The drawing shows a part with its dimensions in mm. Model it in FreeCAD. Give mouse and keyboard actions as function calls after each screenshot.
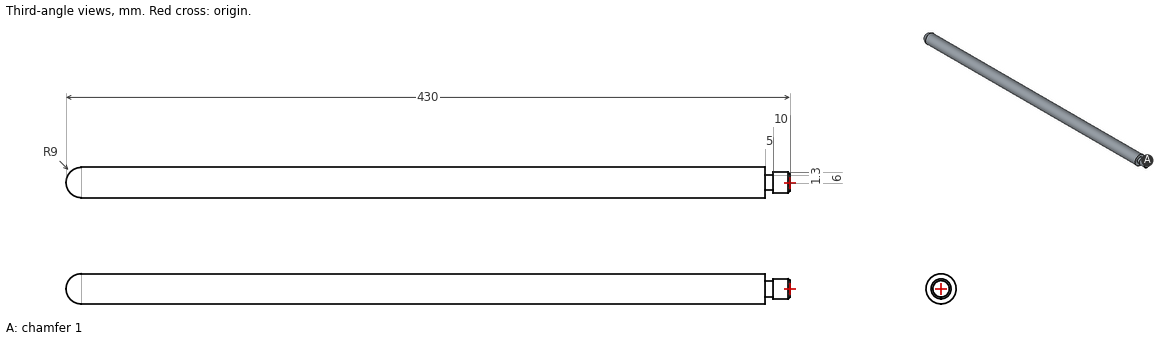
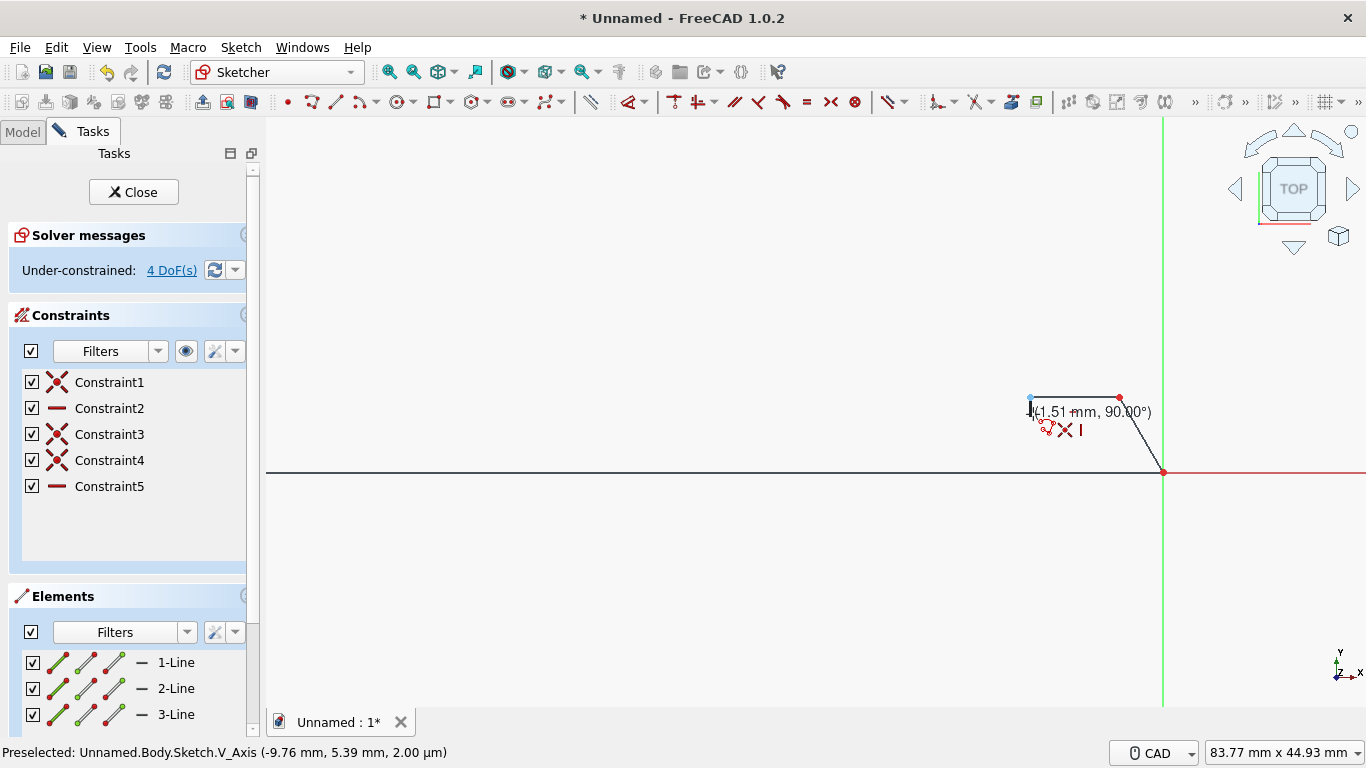
click(1030, 411)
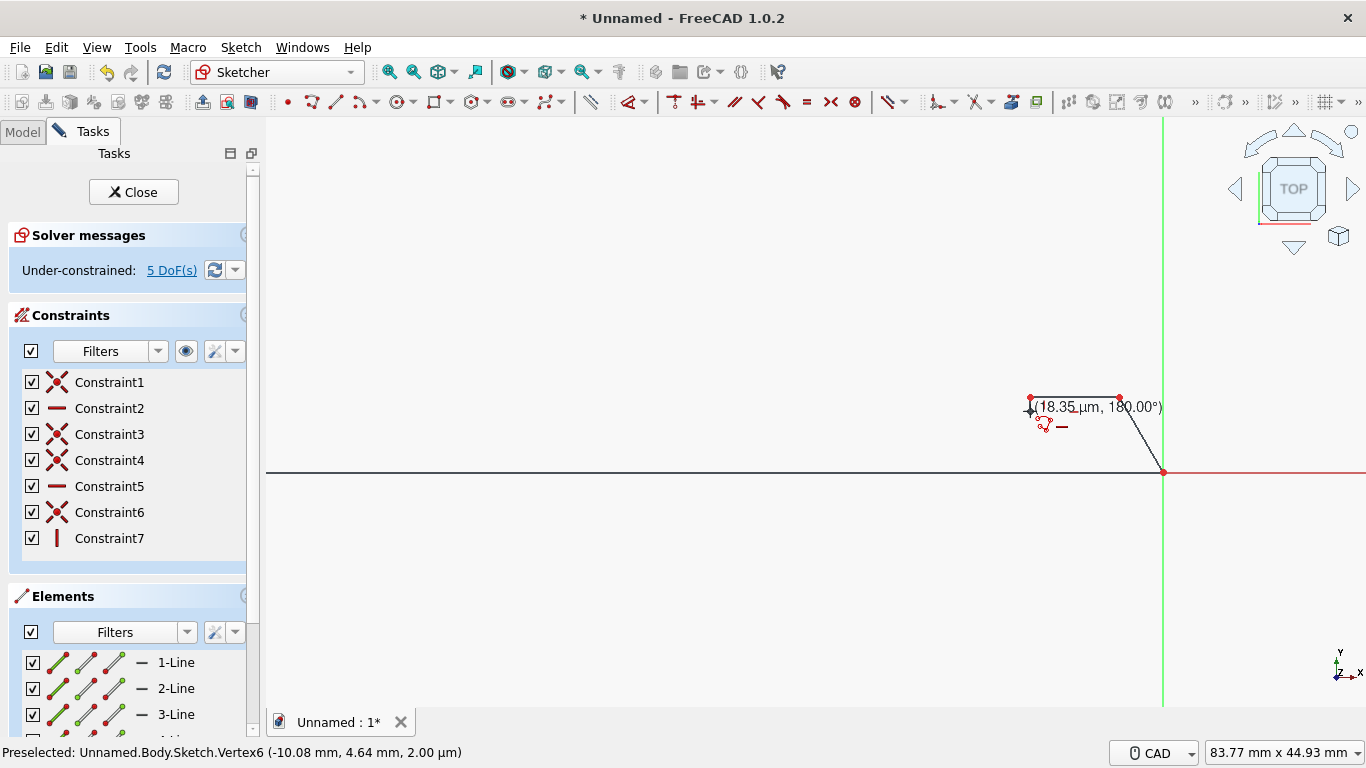
scroll(1047, 412, down, 11)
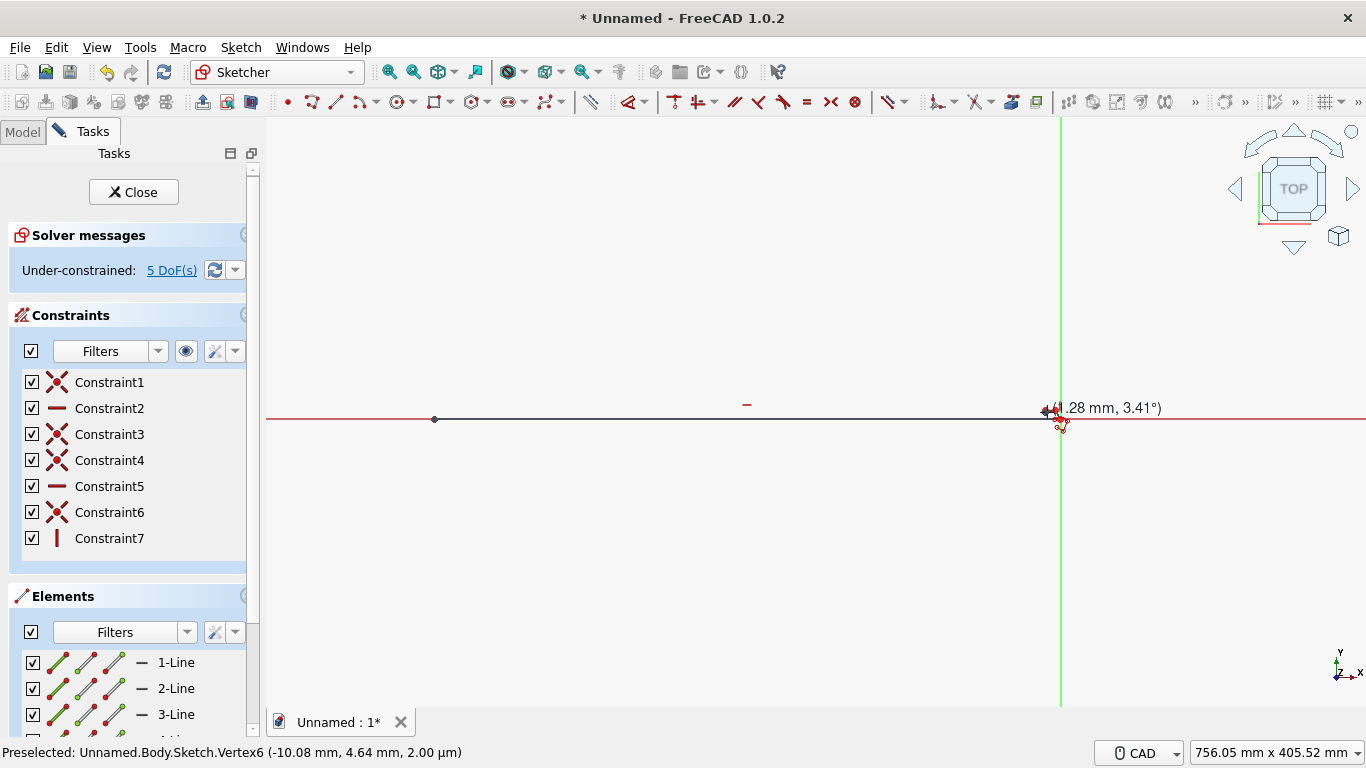
scroll(1039, 412, up, 5)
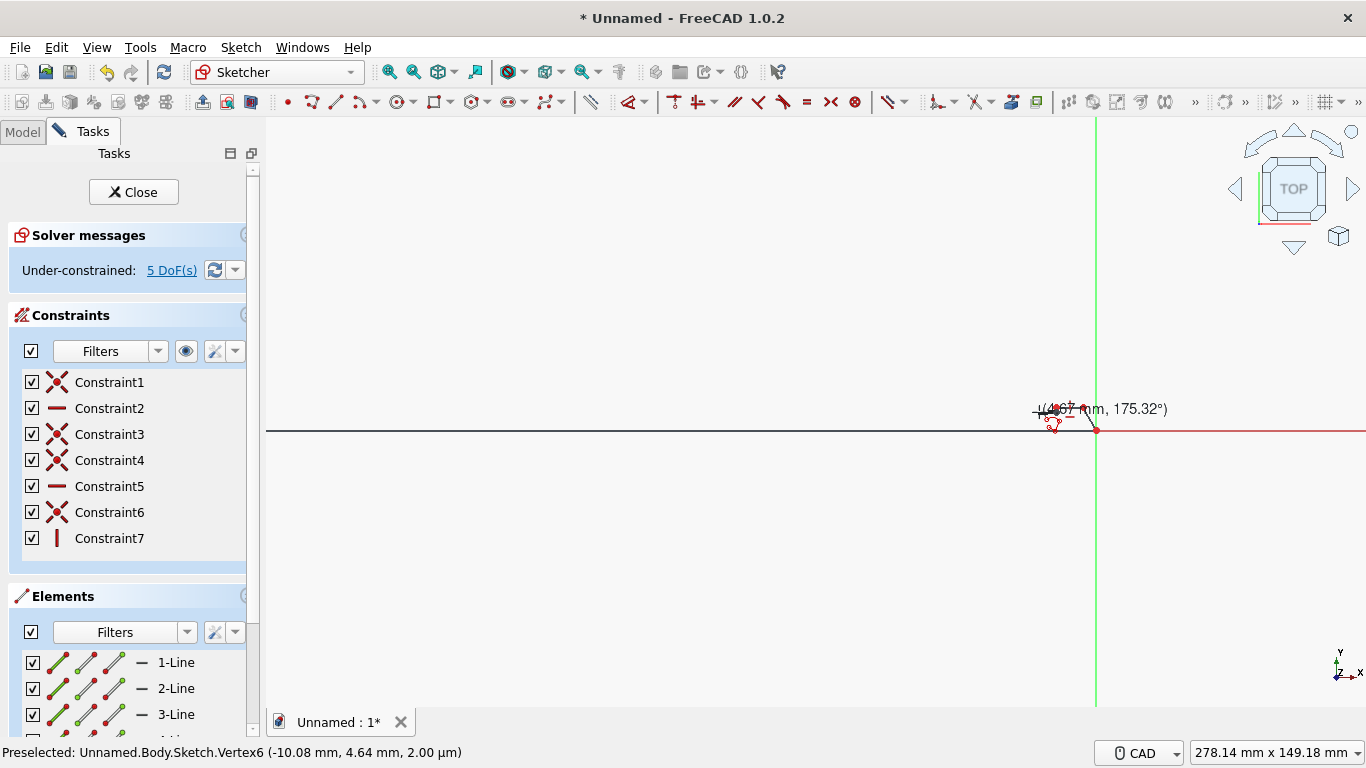
click(1037, 412)
click(1037, 395)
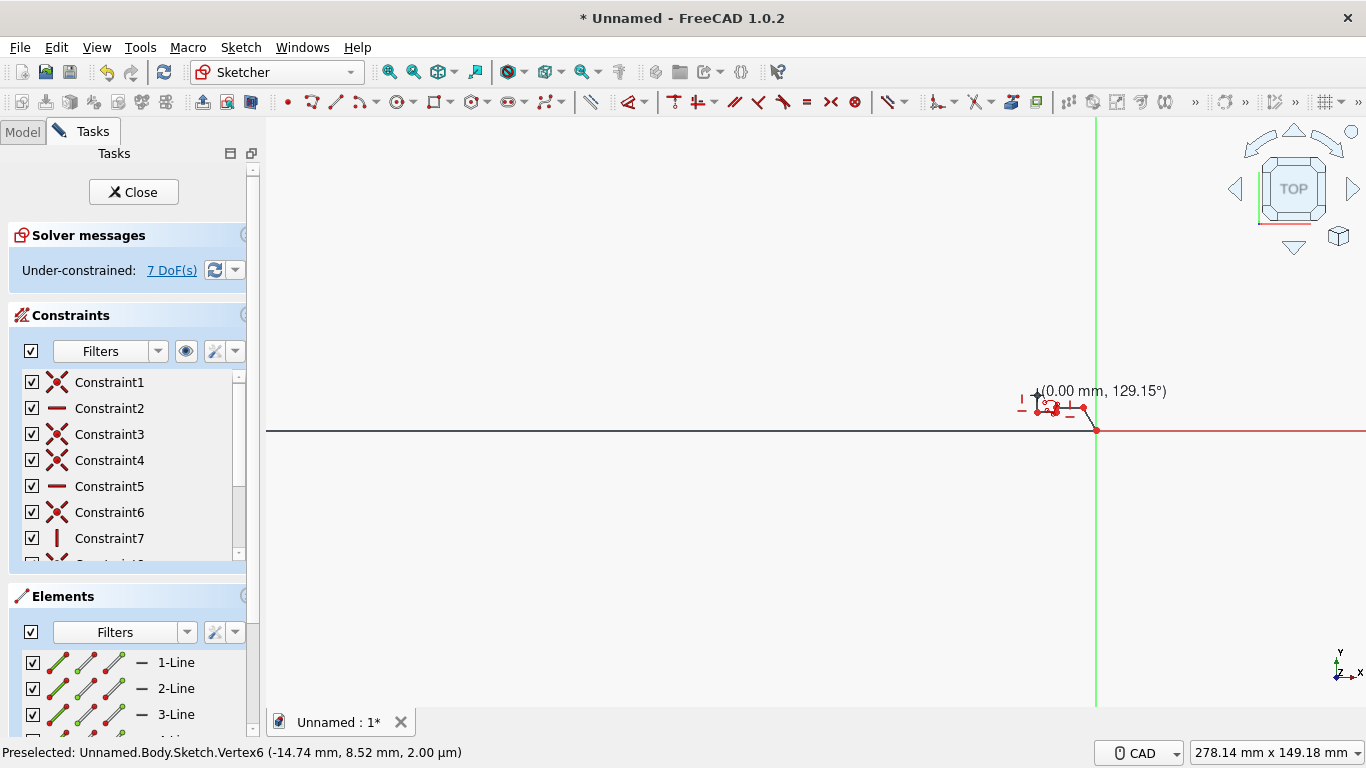
scroll(1039, 411, down, 5)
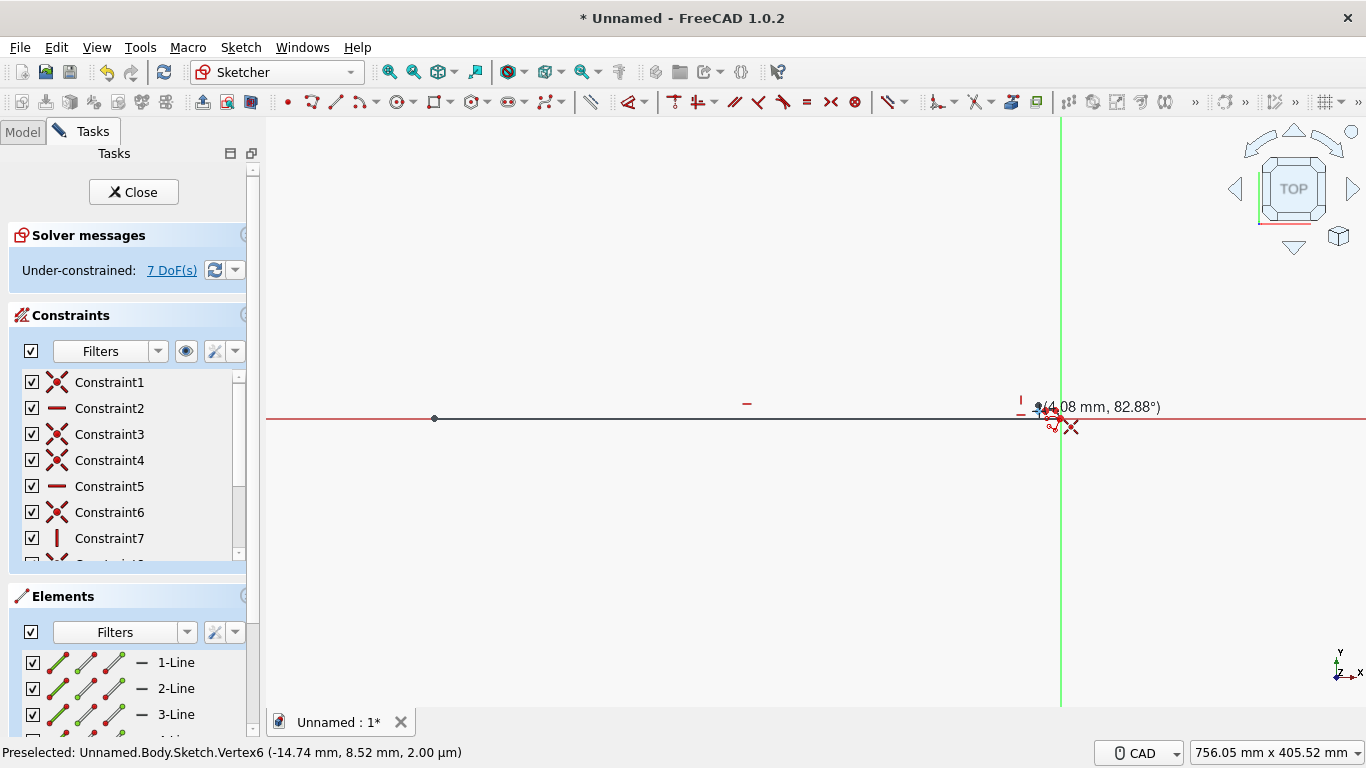
click(448, 405)
right_click(448, 405)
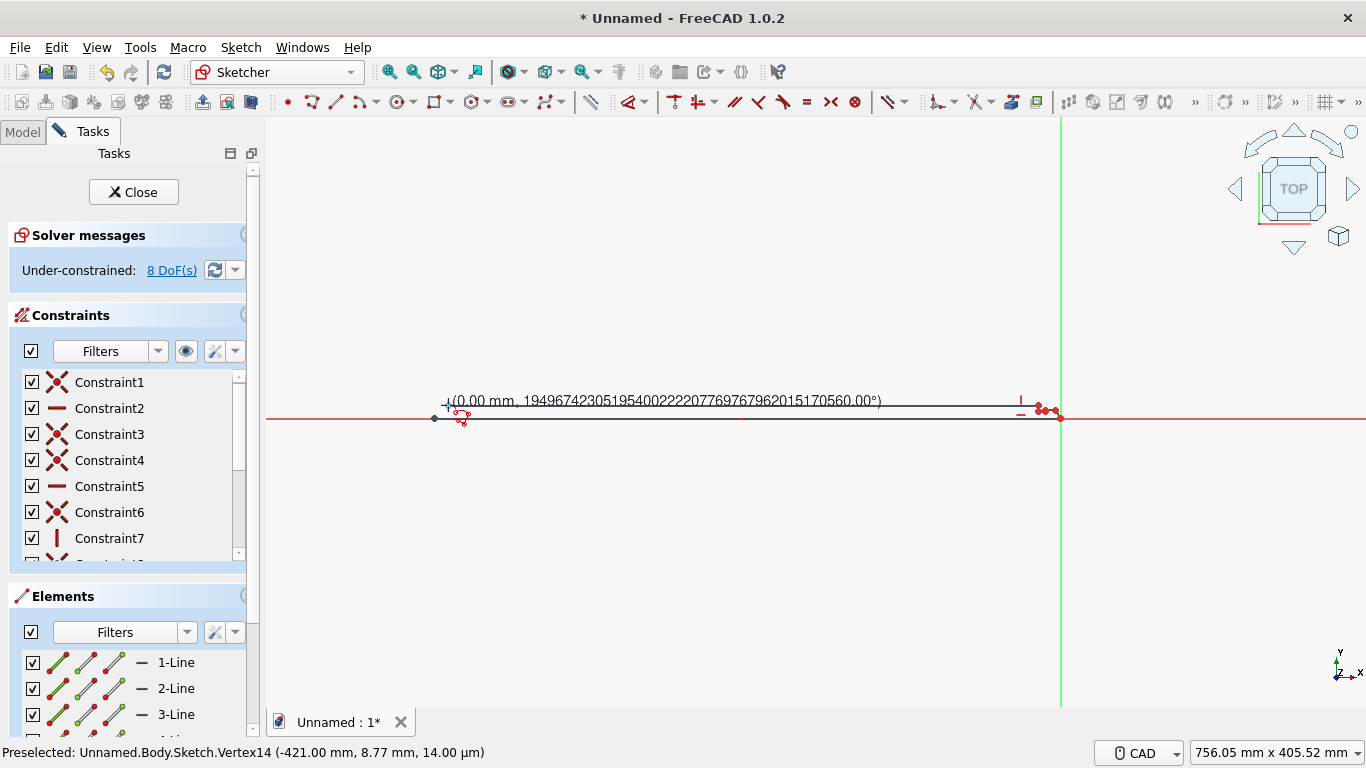
key(g)
key(3)
key(a)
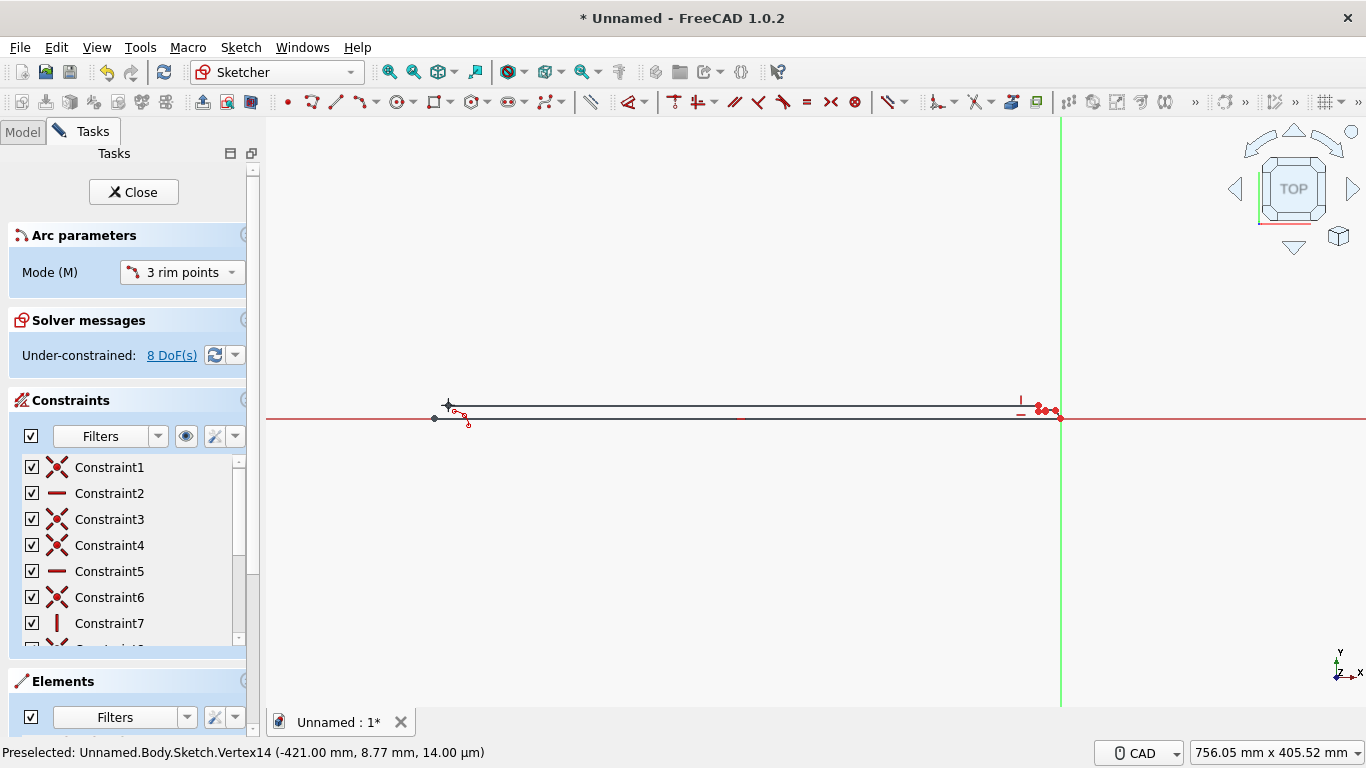
click(448, 406)
click(435, 419)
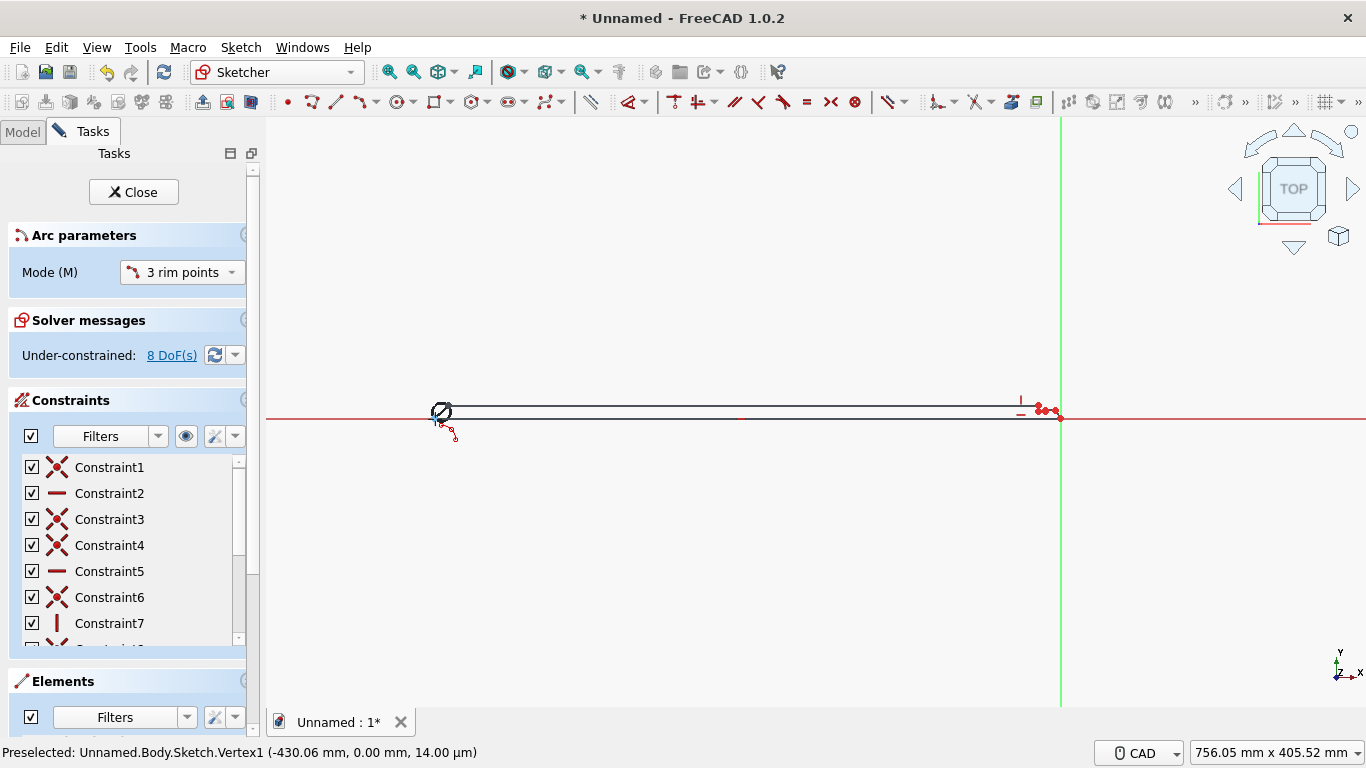
scroll(439, 409, up, 8)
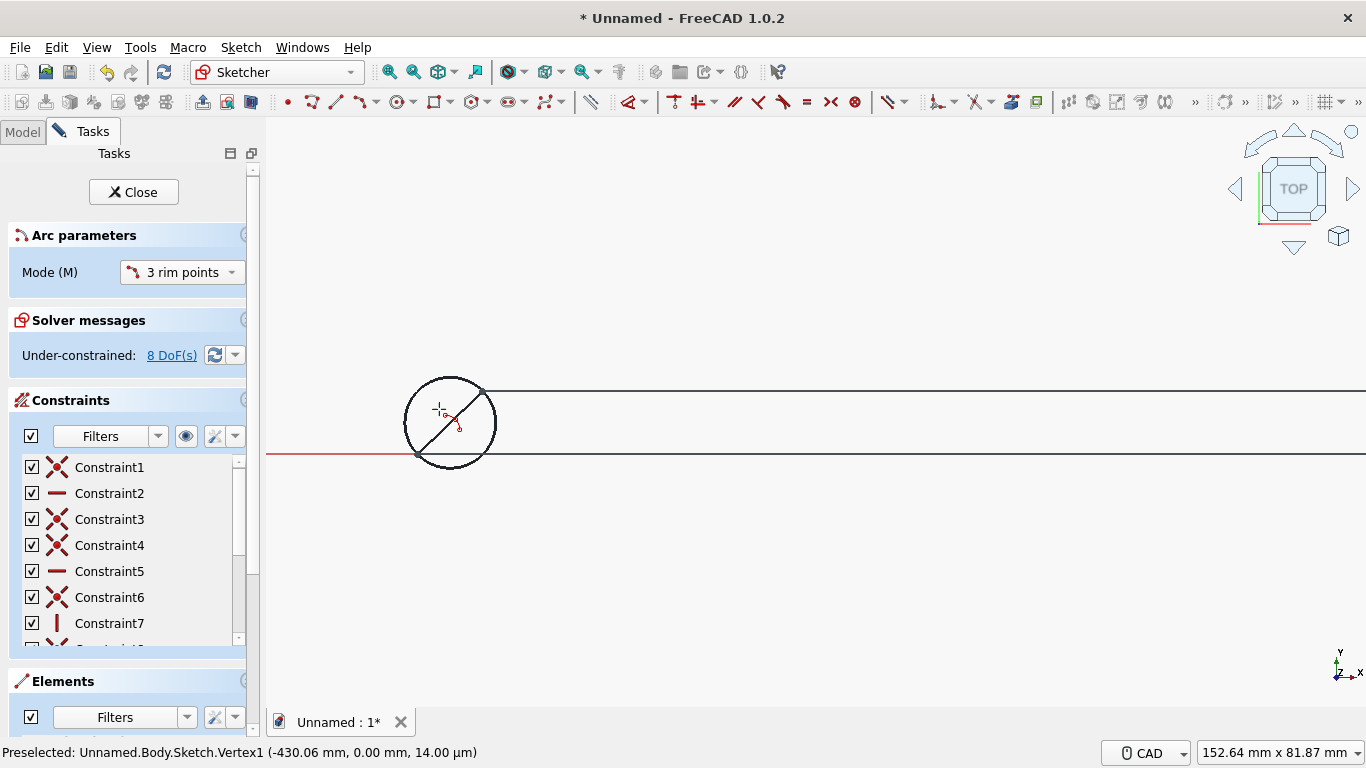
click(437, 409)
key(Escape)